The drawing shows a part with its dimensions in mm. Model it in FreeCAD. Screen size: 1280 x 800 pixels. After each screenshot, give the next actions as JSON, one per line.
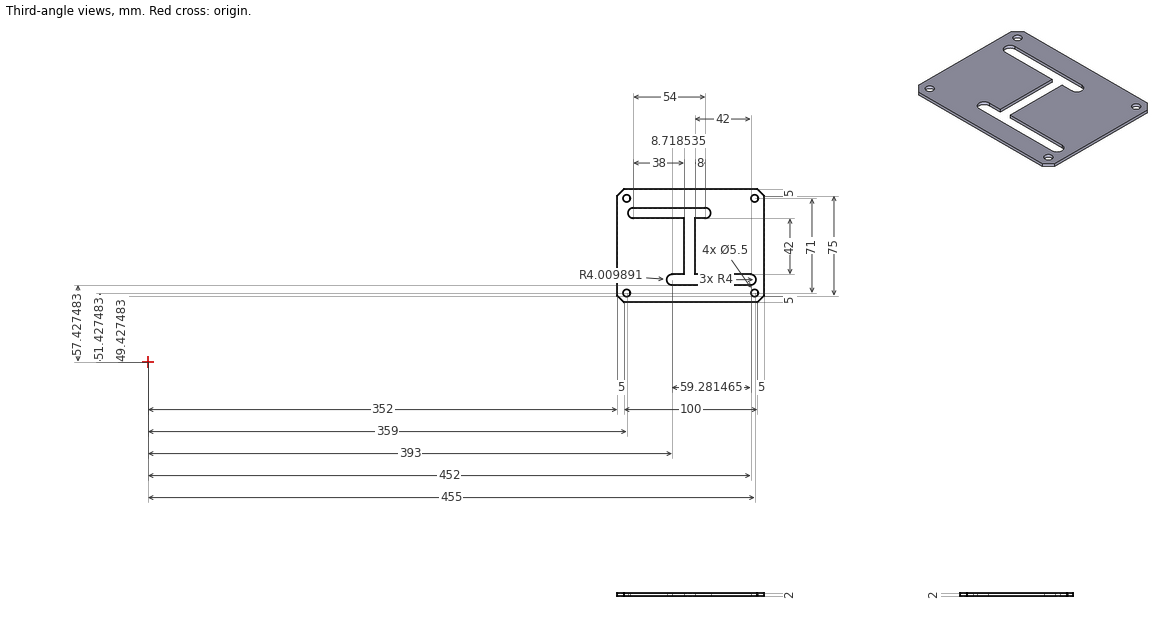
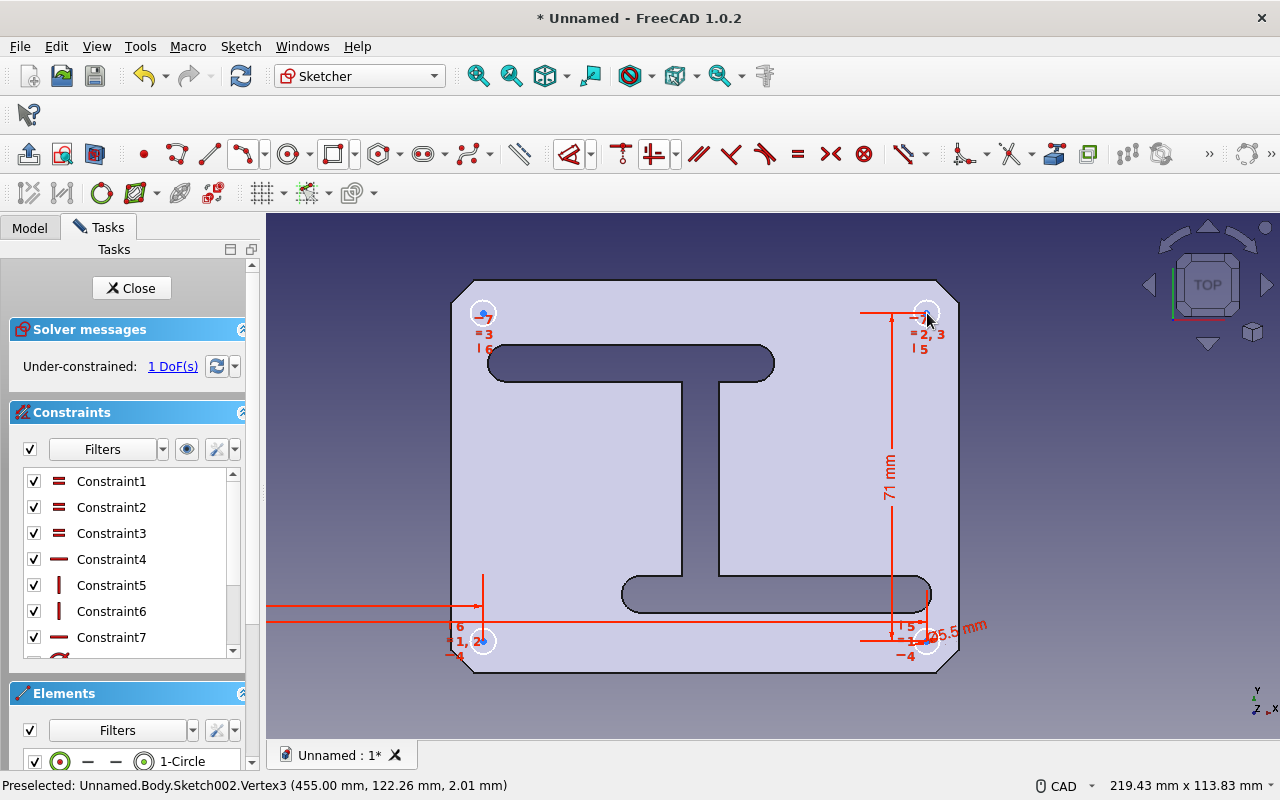
{"action": "left_click", "coordinate": [927, 641]}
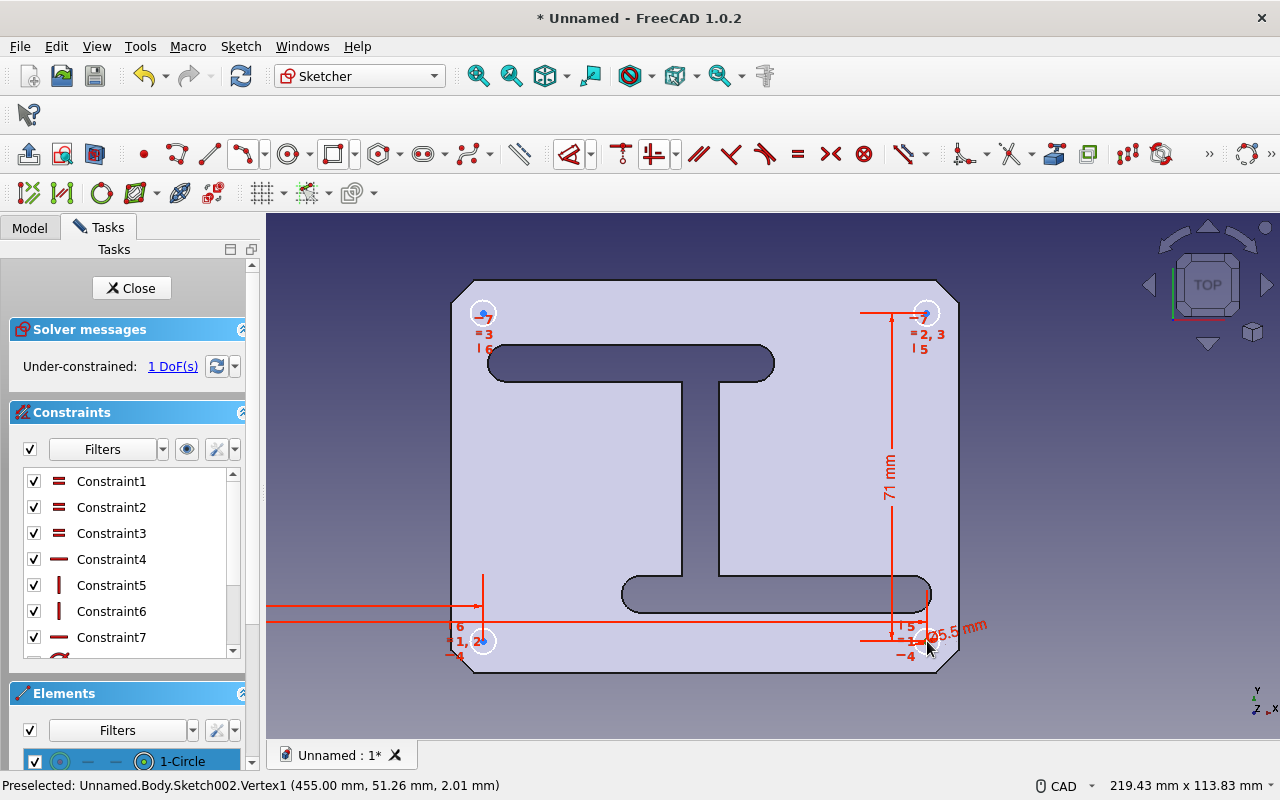
{"action": "key", "text": "i"}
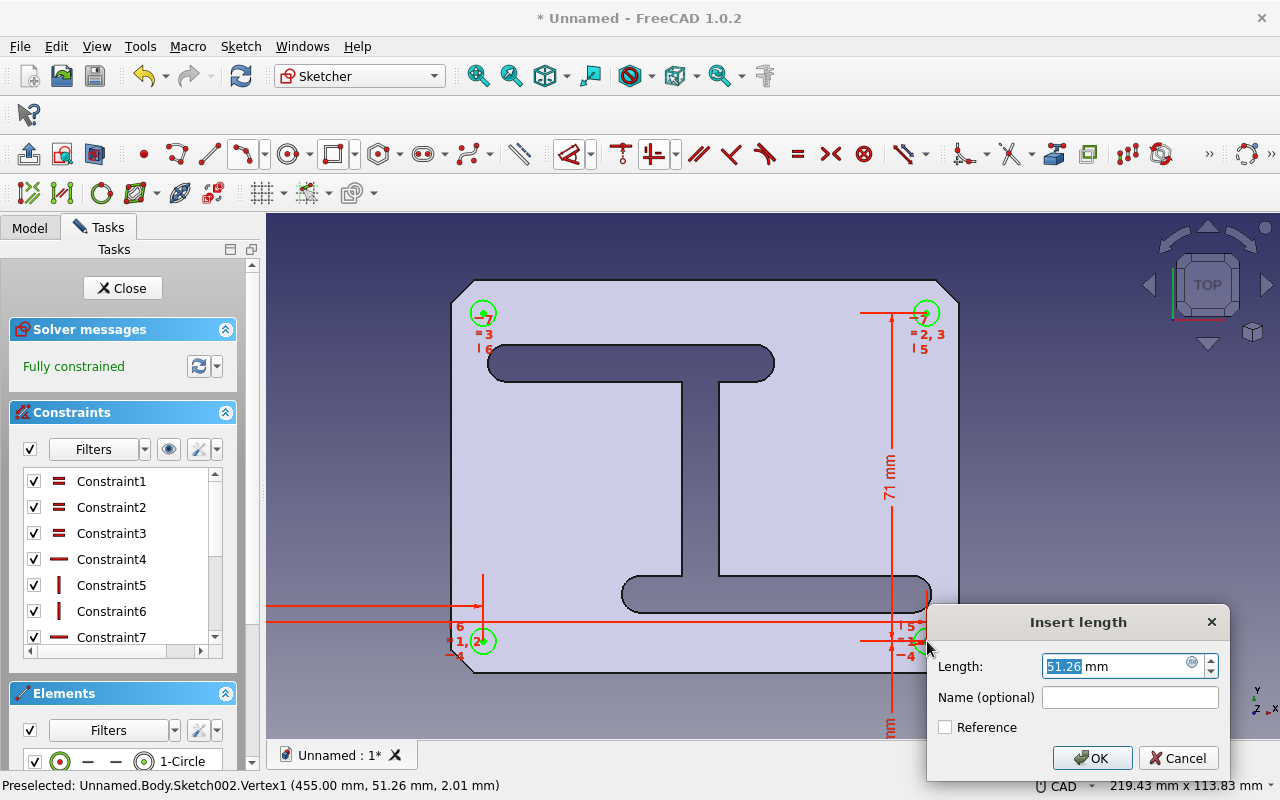
{"action": "type", "text": "51.427483"}
{"action": "key", "text": "Return"}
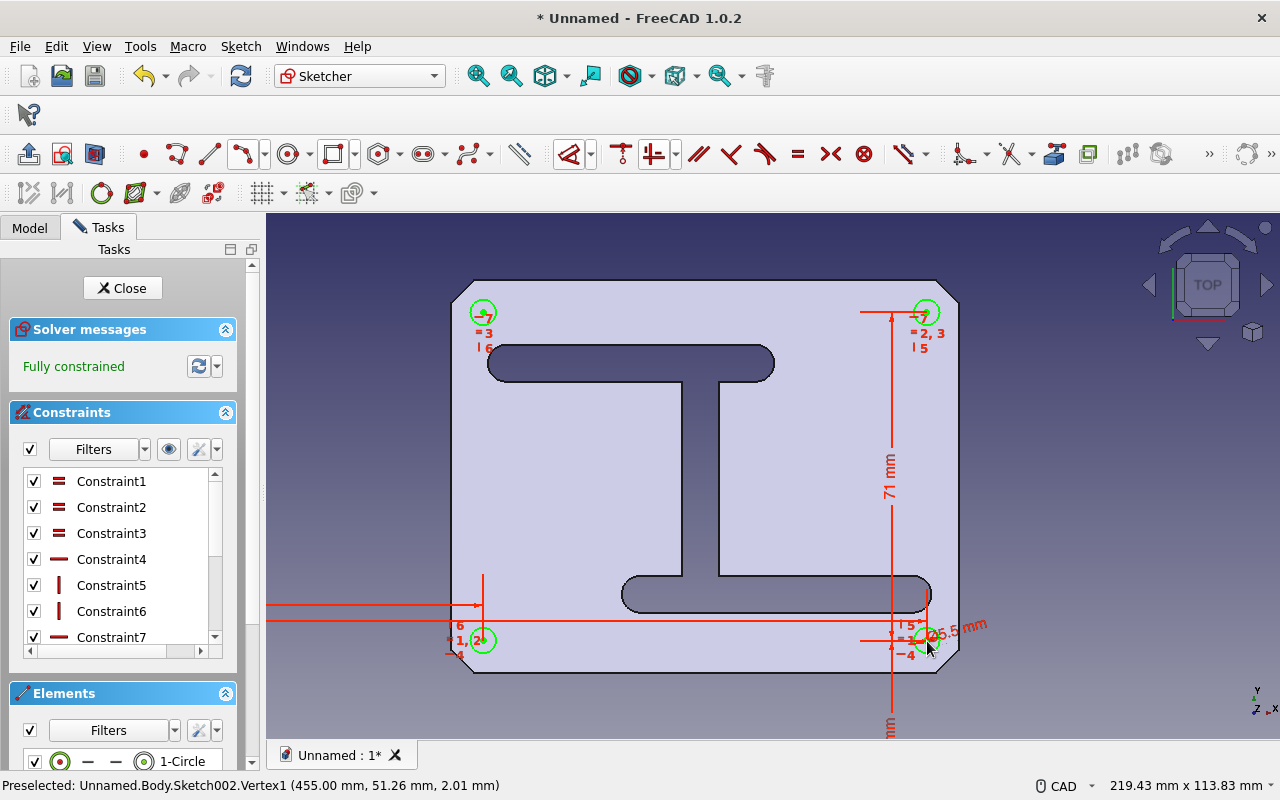
{"action": "left_click", "coordinate": [123, 288]}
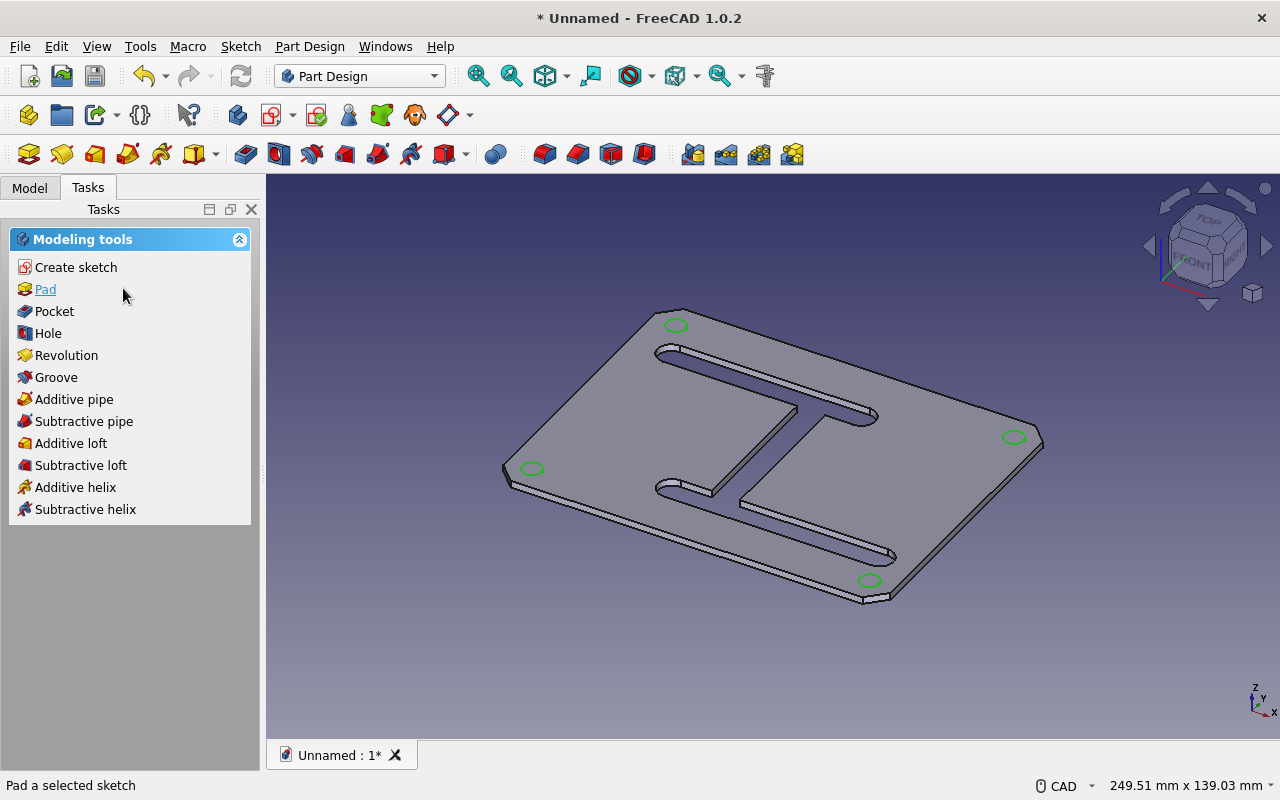
{"action": "left_click", "coordinate": [246, 154]}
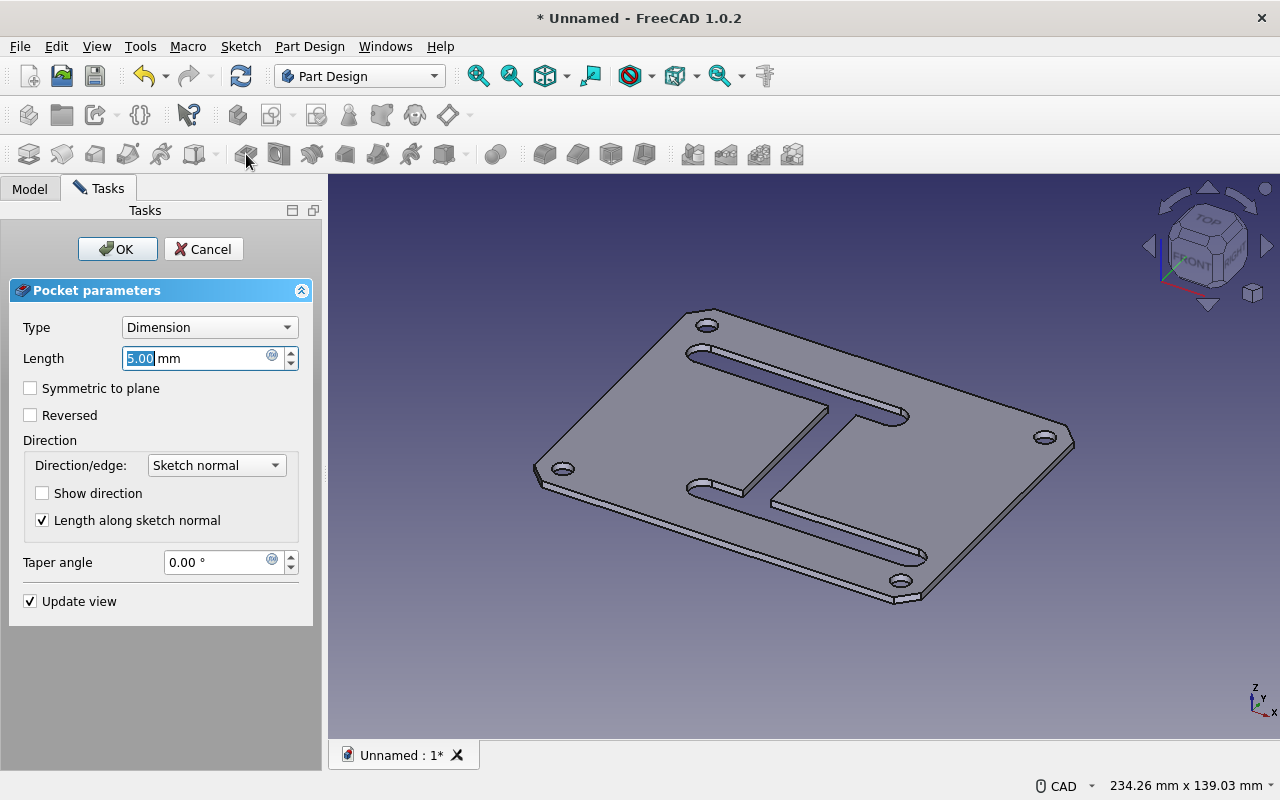
{"action": "type", "text": "2"}
{"action": "key", "text": "Tab"}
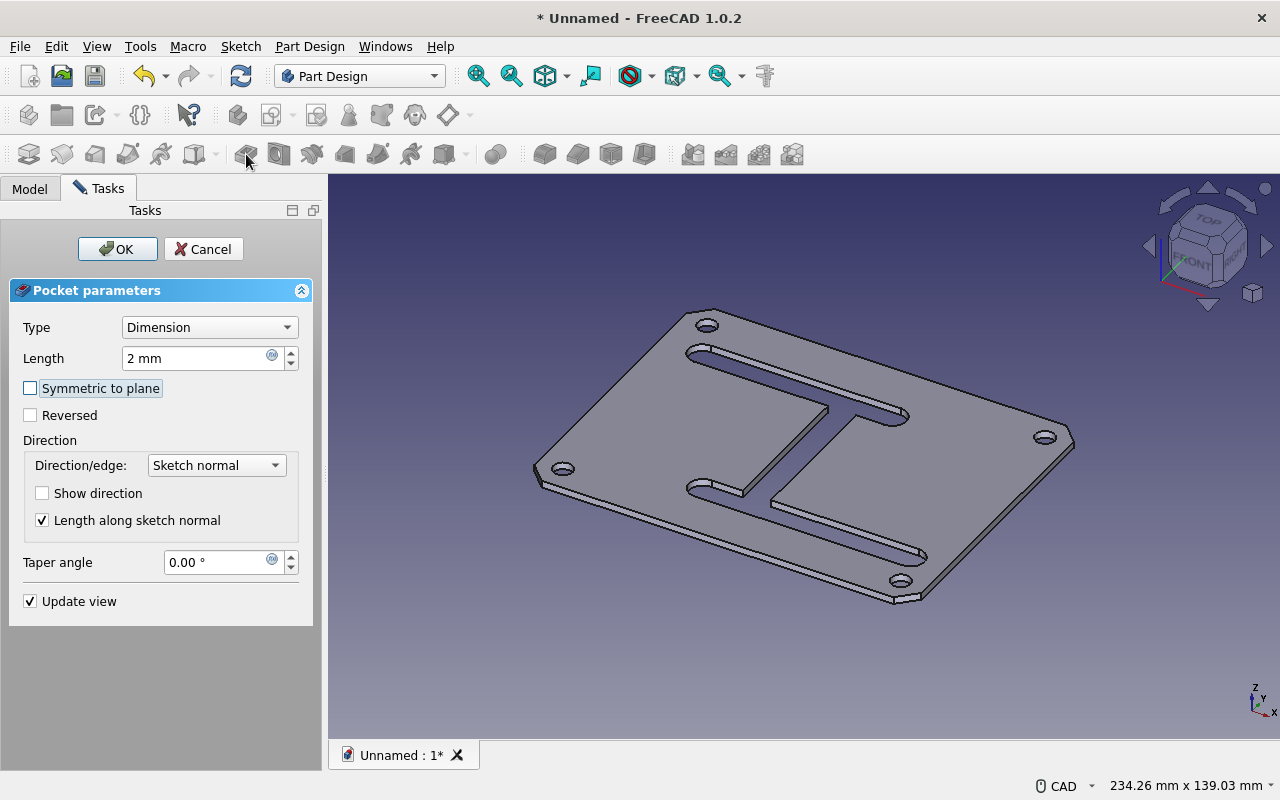
{"action": "left_click", "coordinate": [118, 249]}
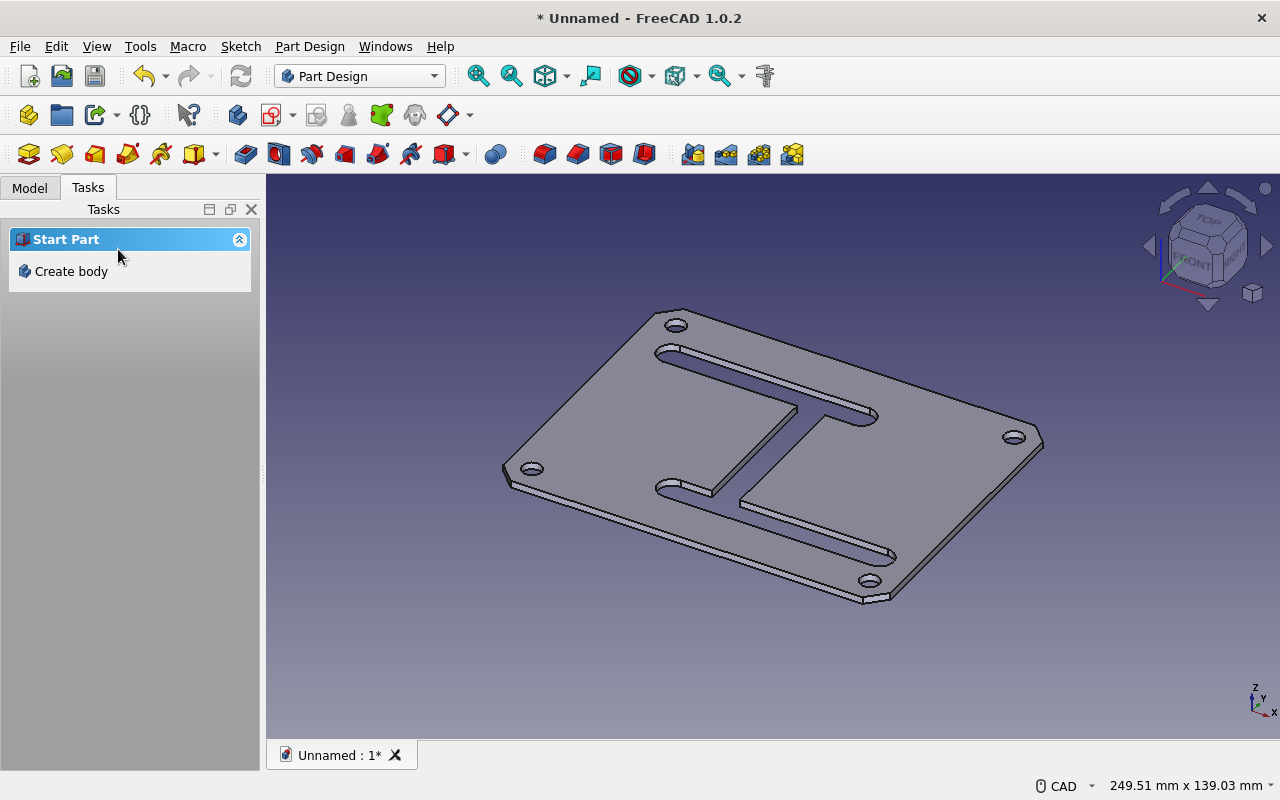
{"action": "key", "text": "0"}